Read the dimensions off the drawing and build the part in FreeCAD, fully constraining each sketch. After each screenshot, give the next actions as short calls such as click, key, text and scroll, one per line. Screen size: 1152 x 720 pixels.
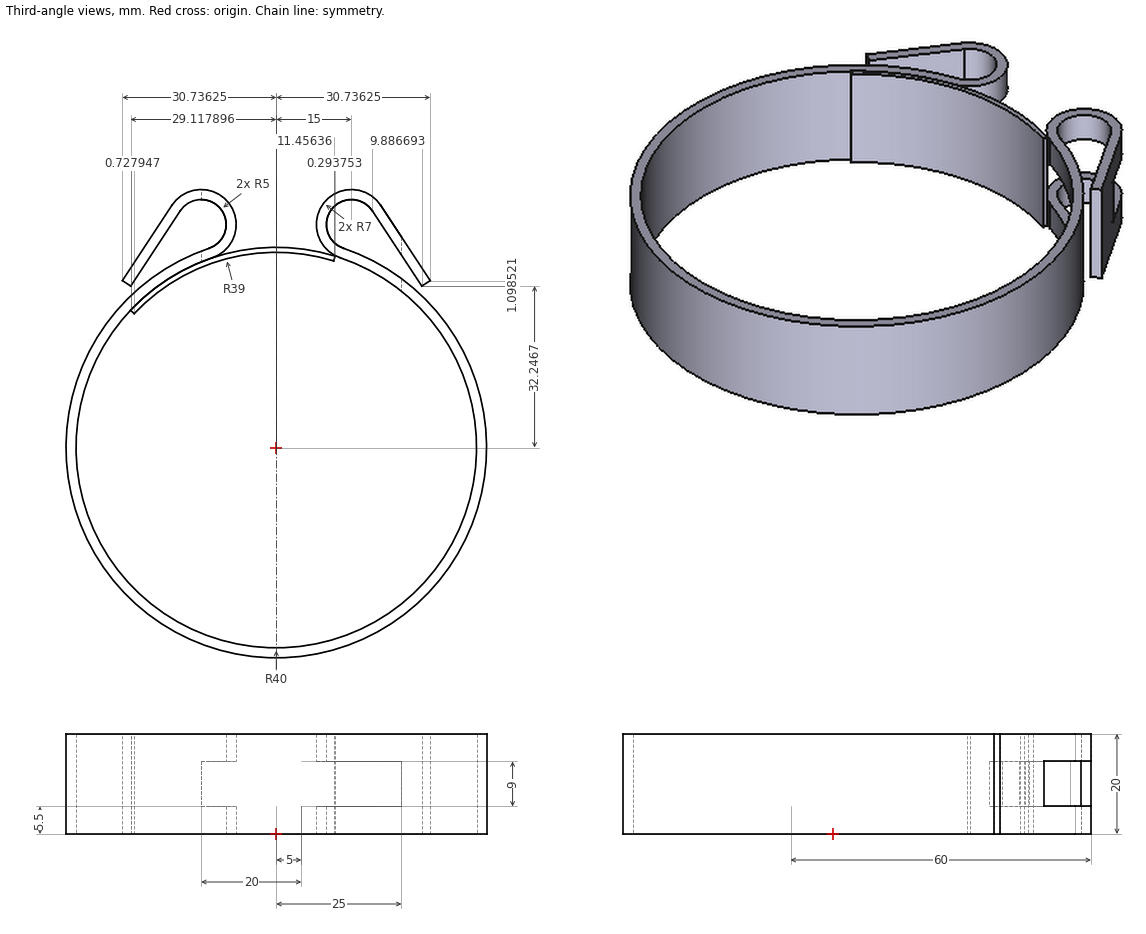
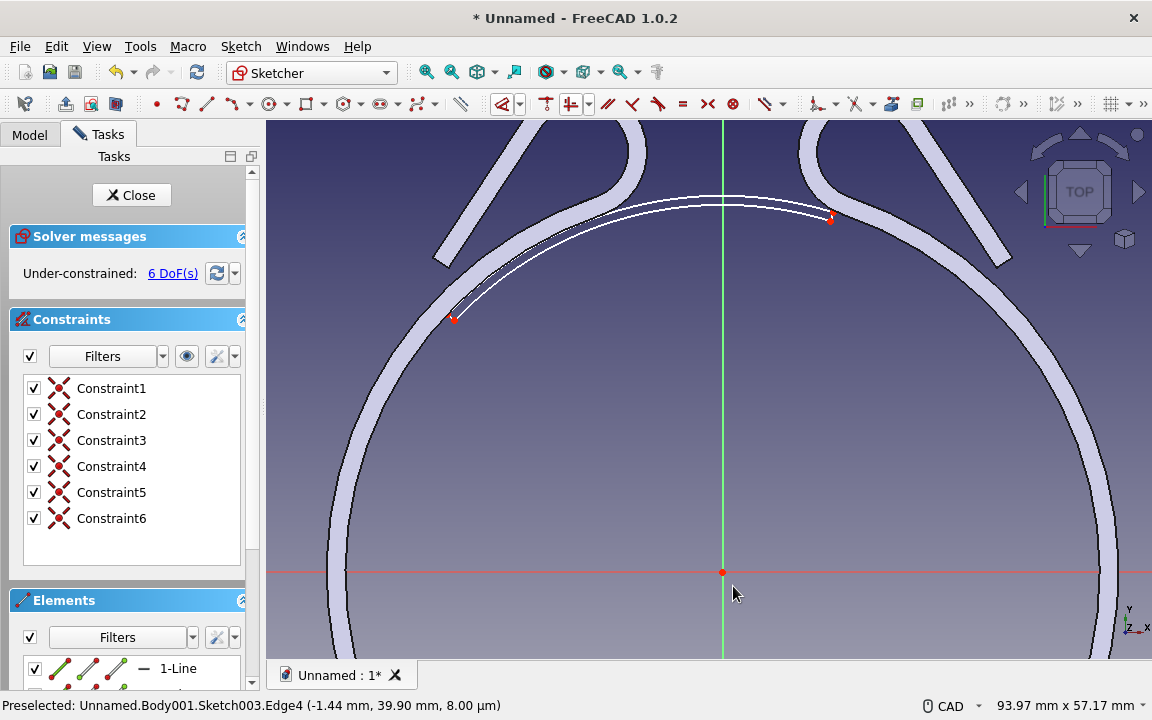
scroll(710, 205, up, 3)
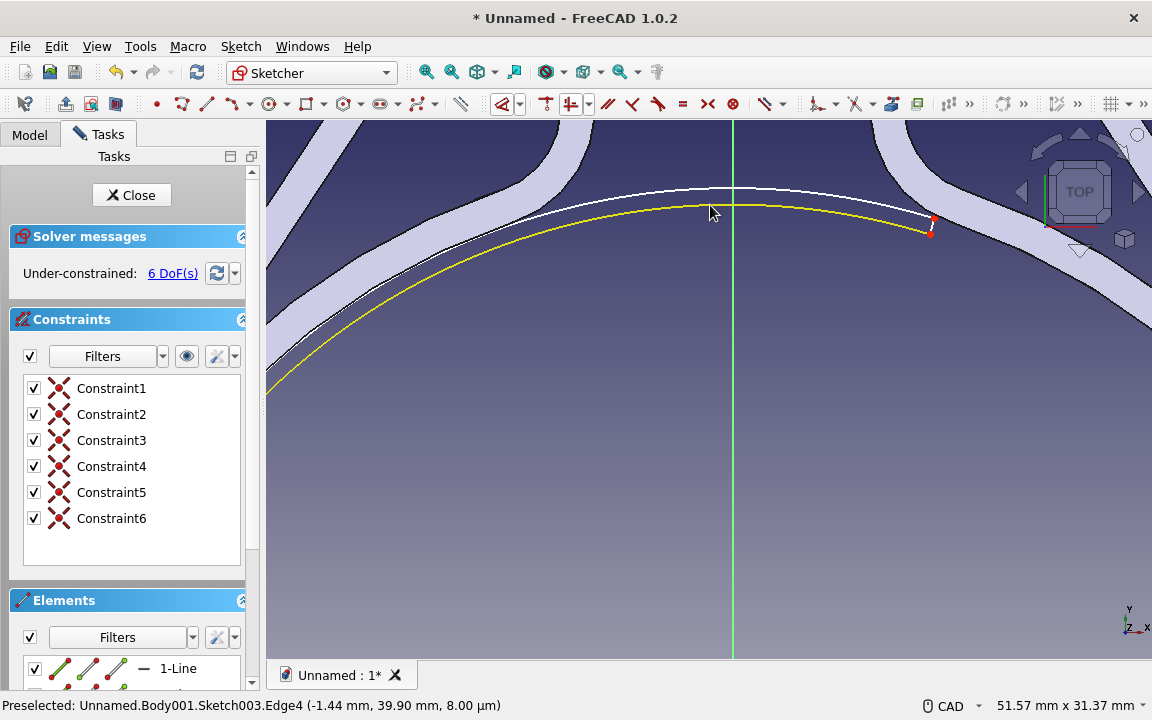
click(709, 205)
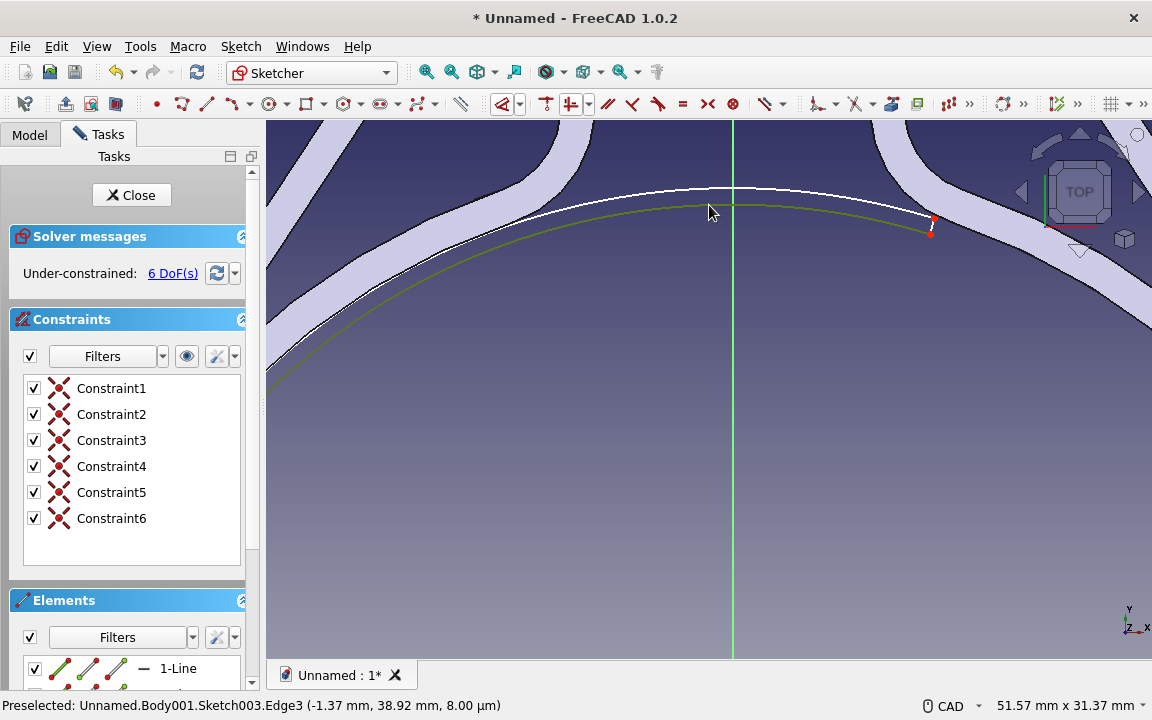
click(520, 104)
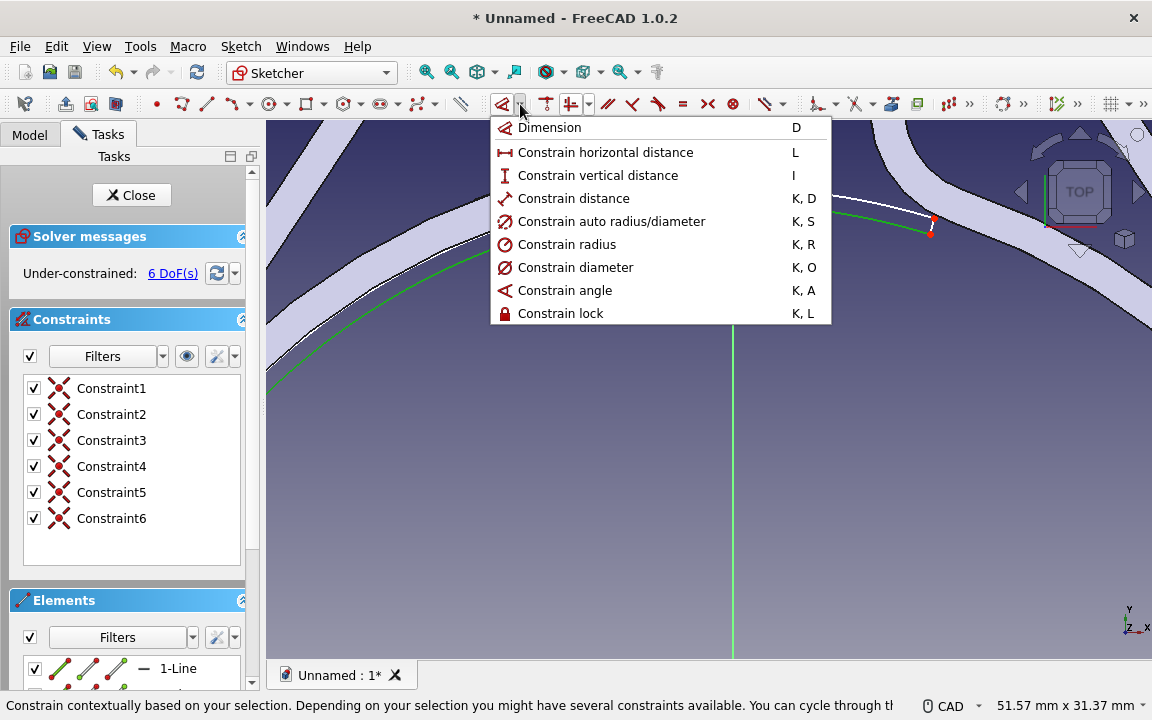
click(661, 244)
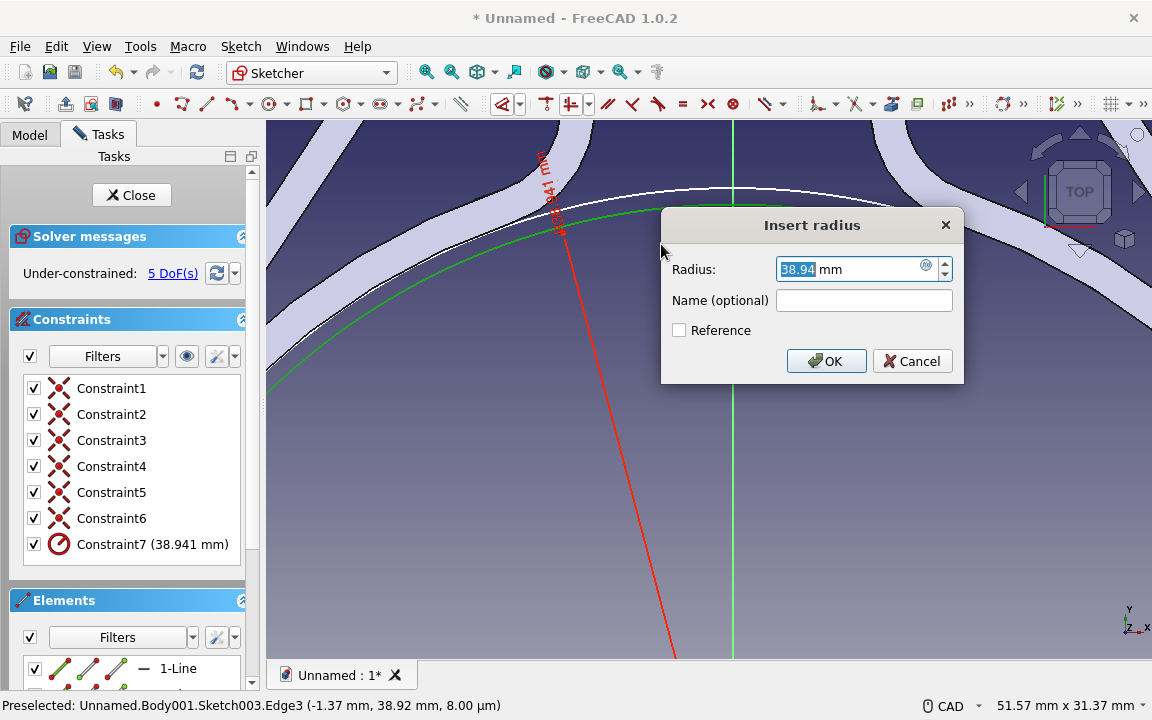
text(39)
key(Return)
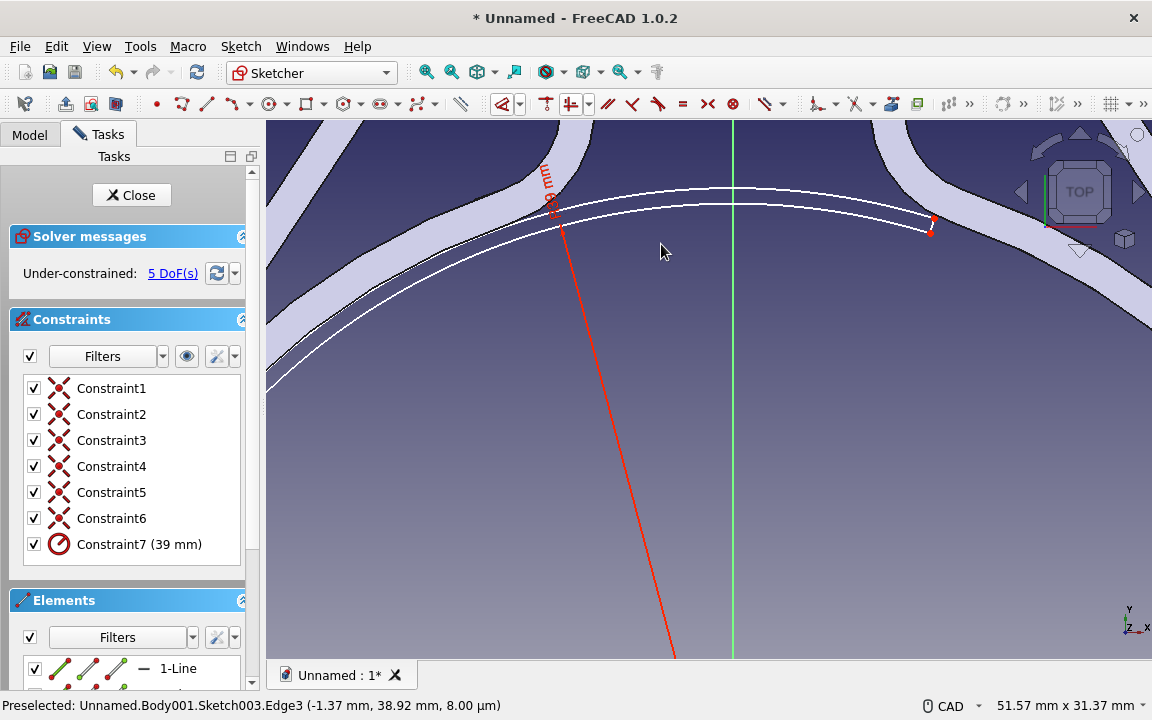
click(708, 189)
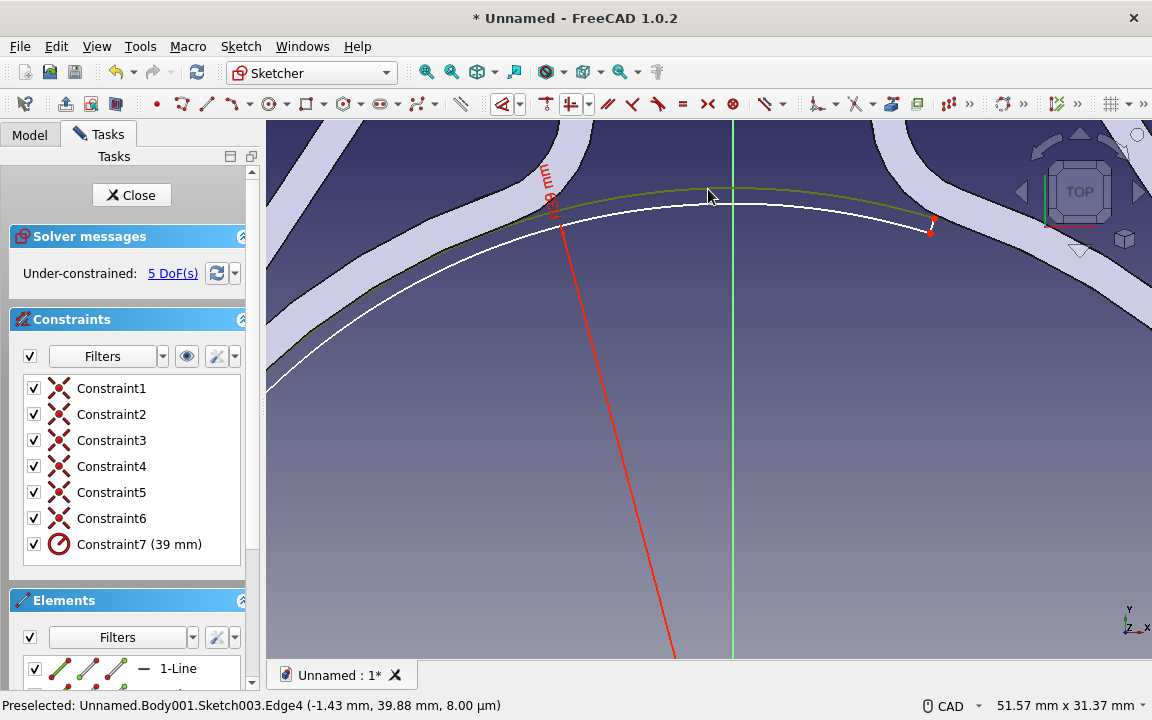
key(k)
key(r)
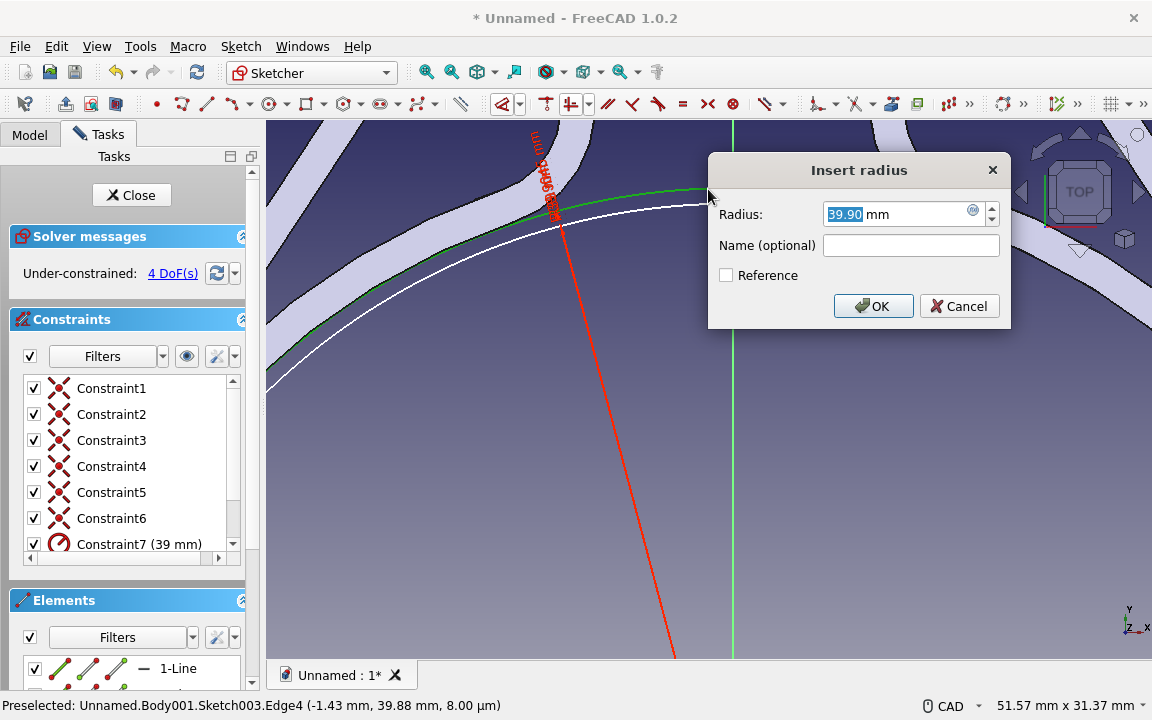
text(40)
key(Return)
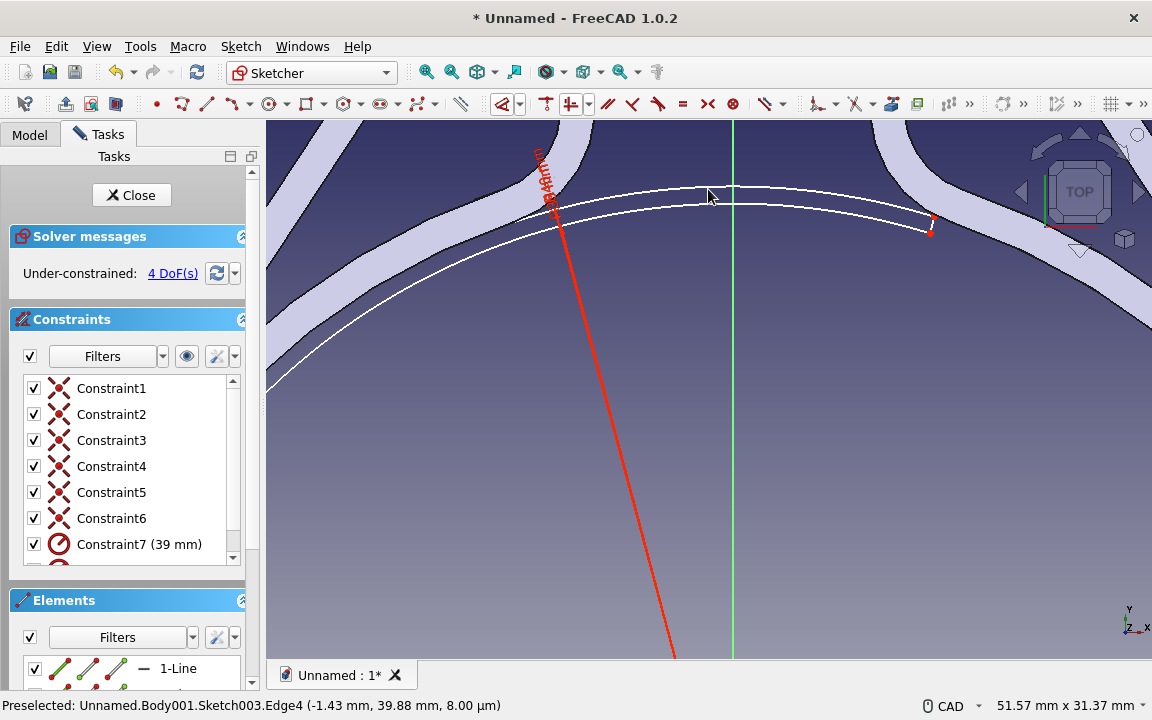
click(930, 233)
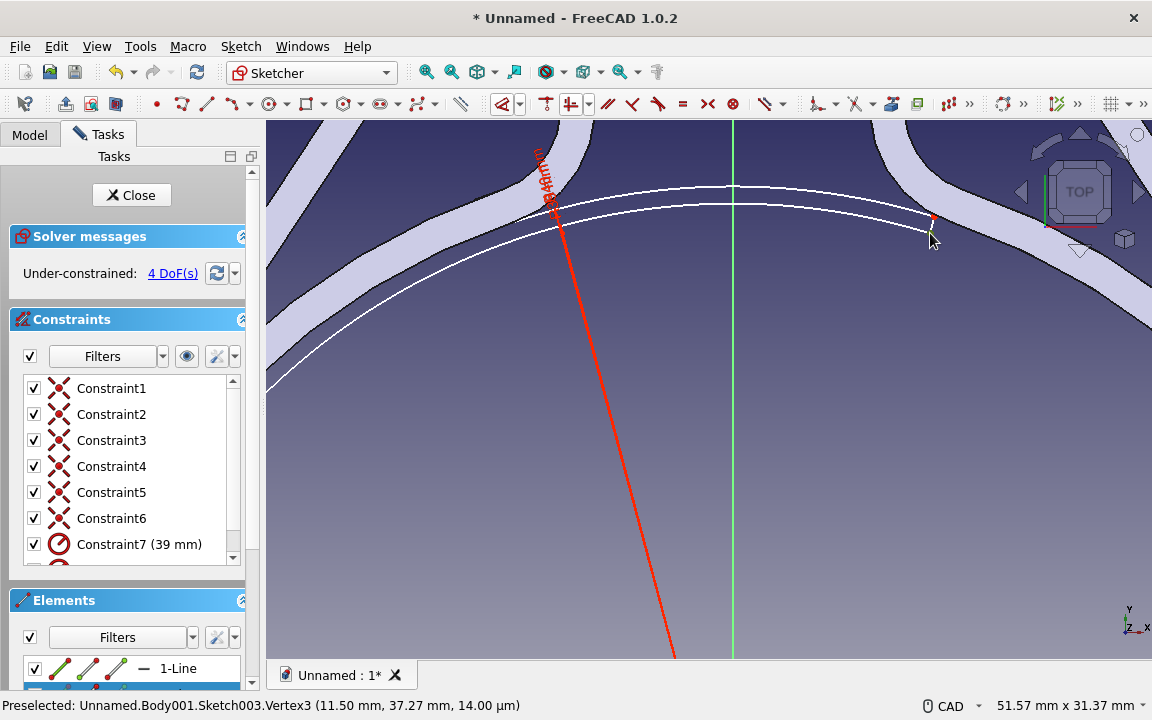
key(l)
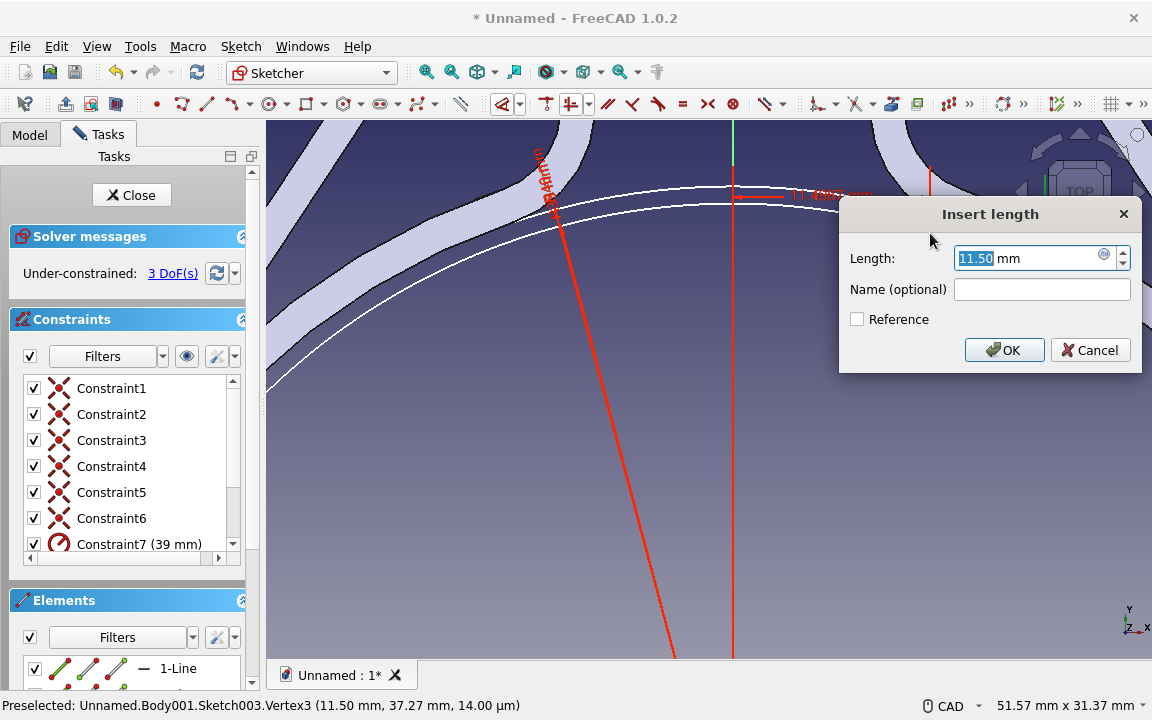
text(11.45636)
key(Return)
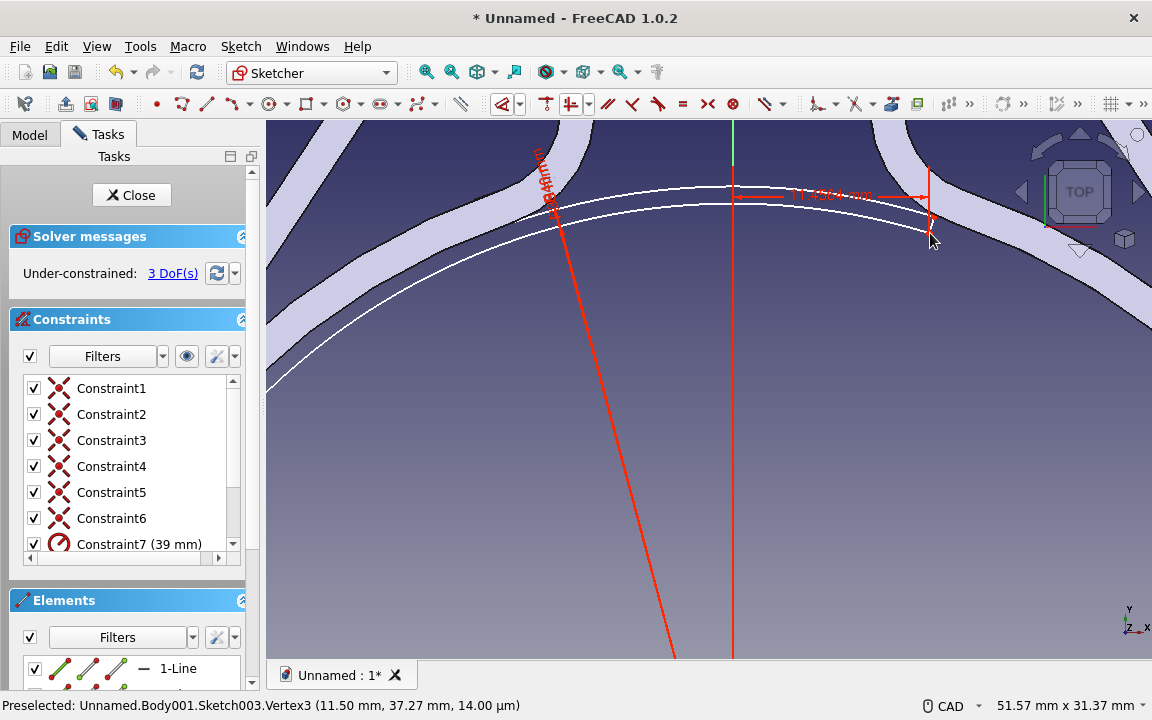
scroll(710, 205, down, 3)